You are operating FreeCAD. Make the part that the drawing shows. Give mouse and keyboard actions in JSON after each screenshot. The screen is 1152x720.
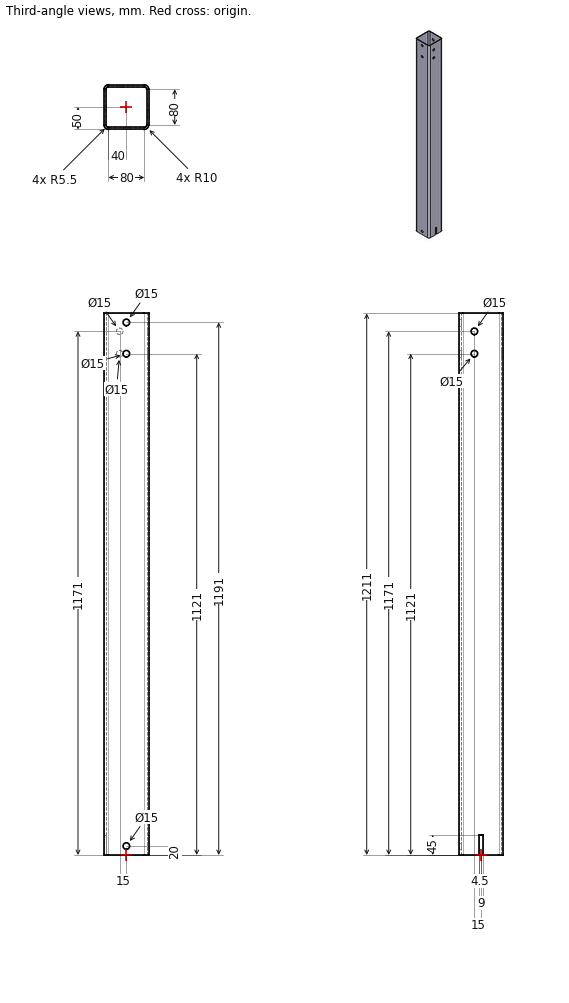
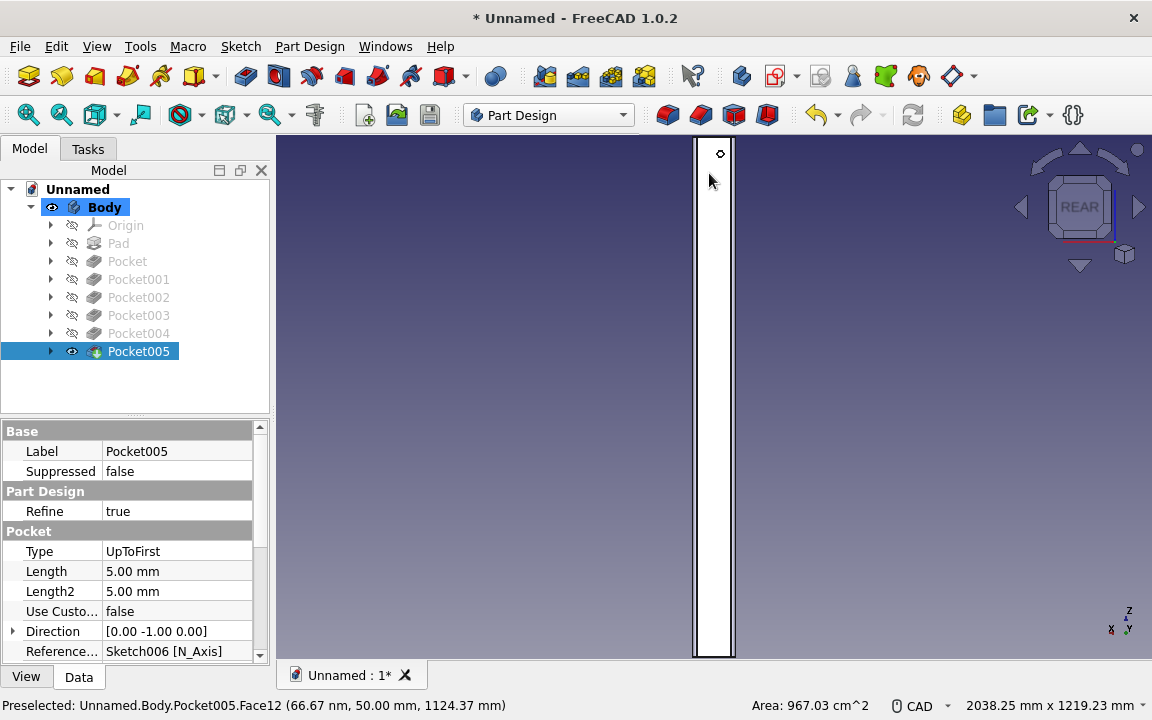
{"action": "left_click", "coordinate": [774, 76]}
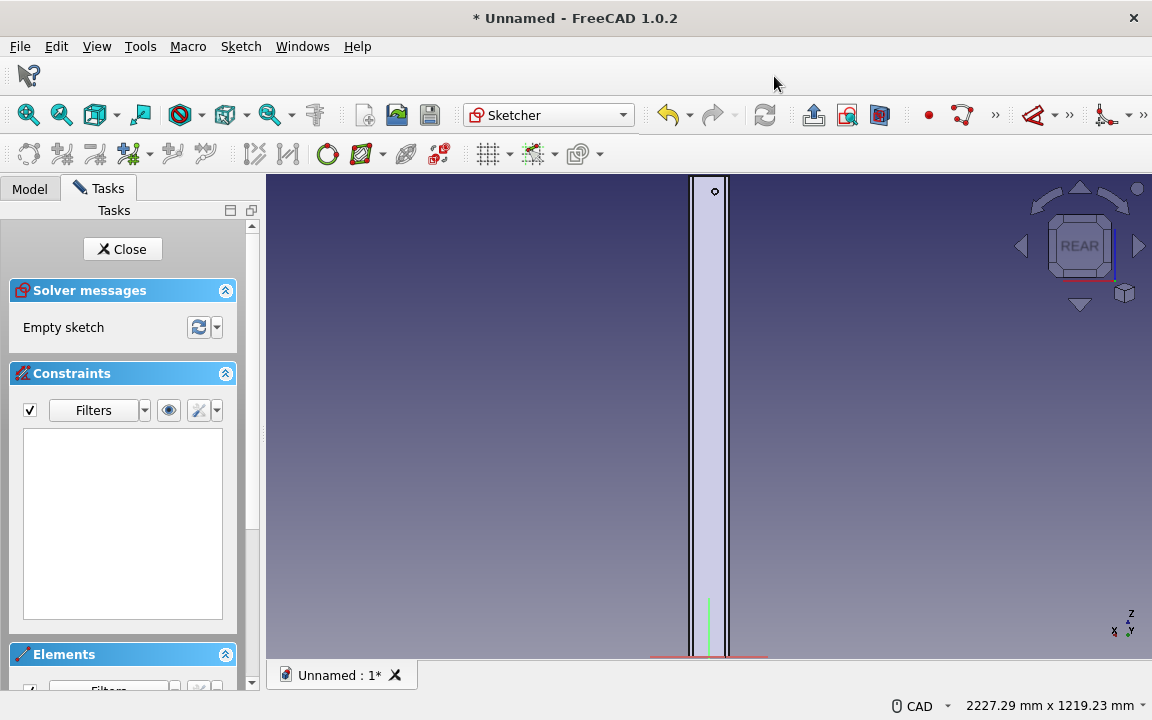
{"action": "scroll", "coordinate": [719, 202], "scroll_direction": "up", "scroll_amount": 15}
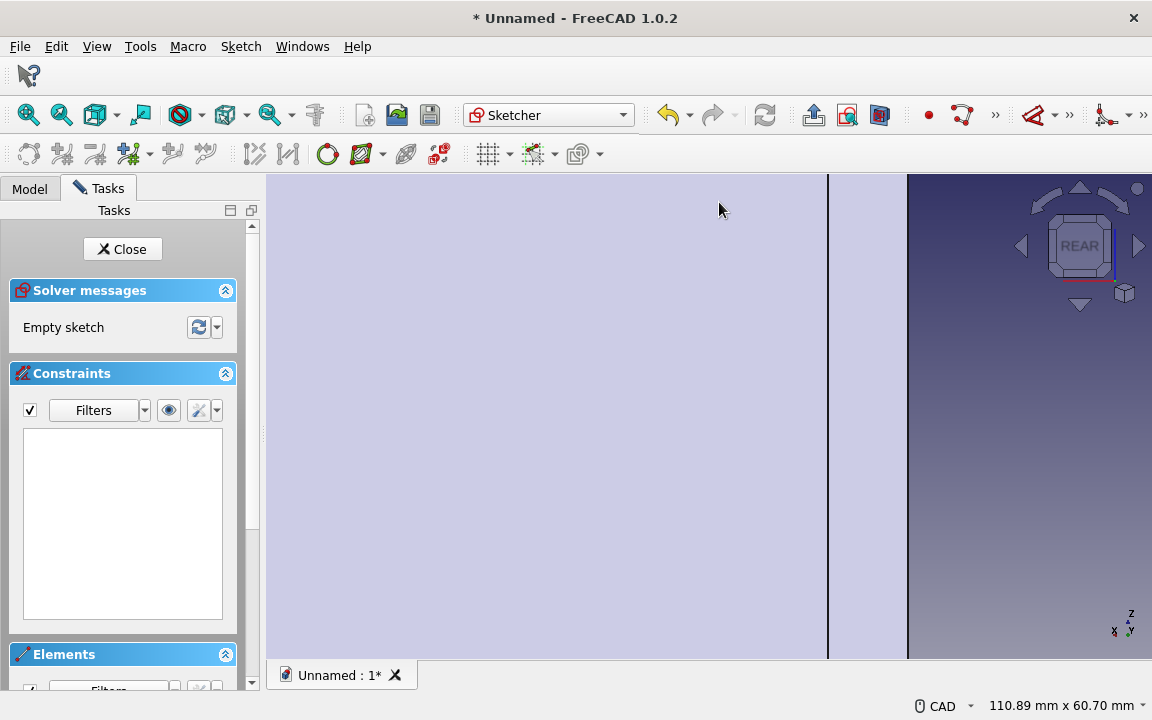
{"action": "scroll", "coordinate": [621, 375], "scroll_direction": "up", "scroll_amount": 5}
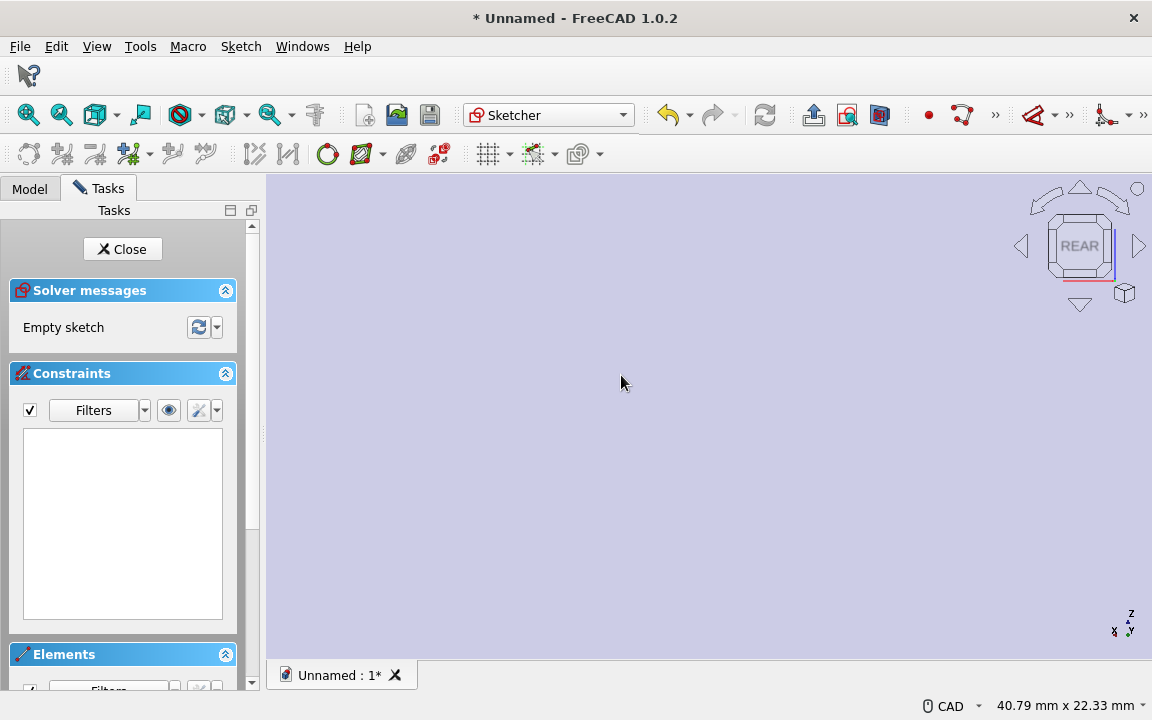
{"action": "key", "text": "g c"}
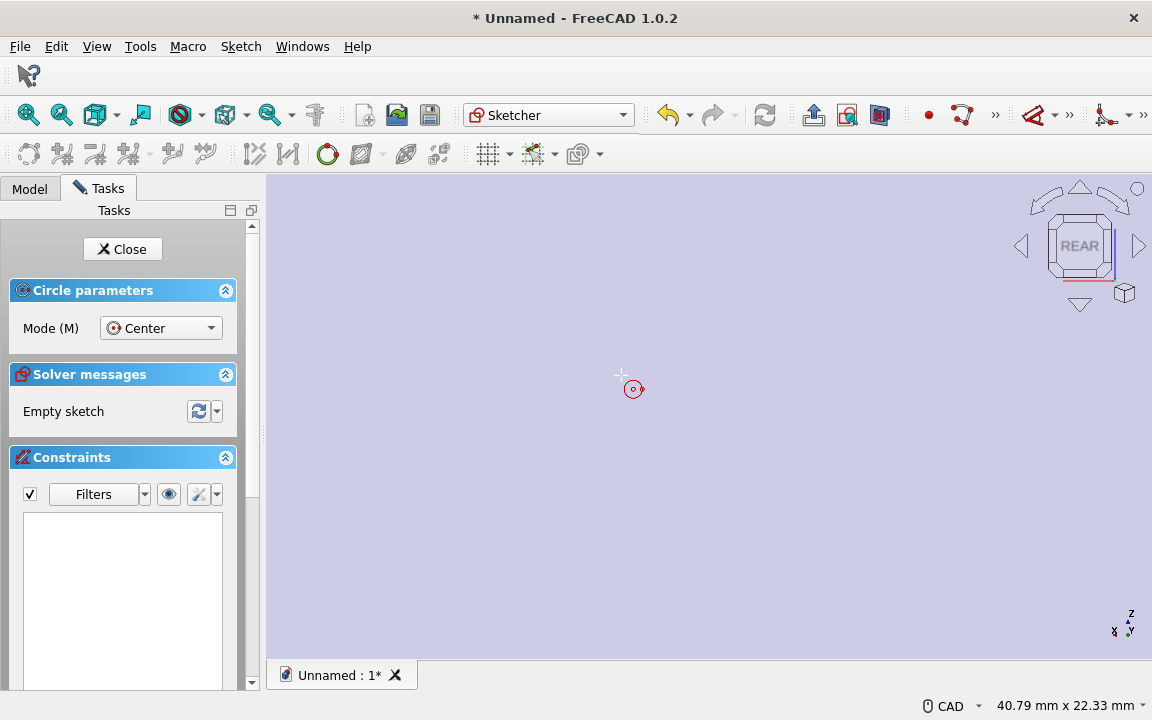
{"action": "left_click", "coordinate": [640, 416]}
{"action": "left_click", "coordinate": [755, 301]}
{"action": "key", "text": "Escape"}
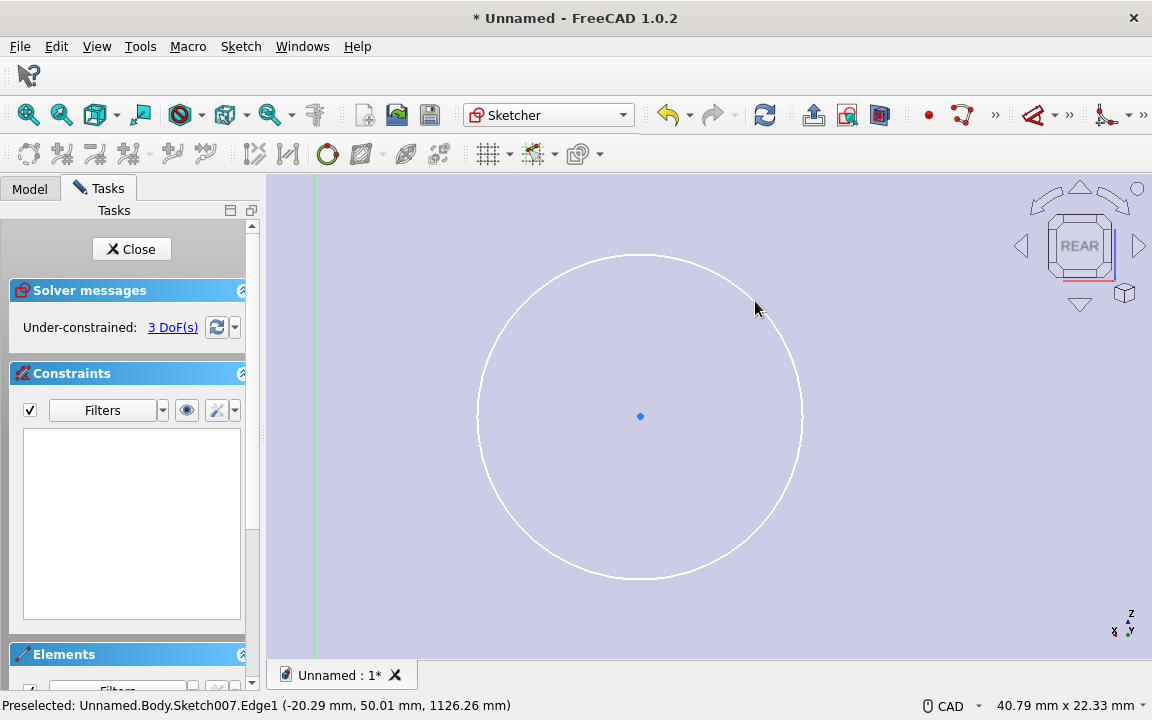
{"action": "key", "text": "d"}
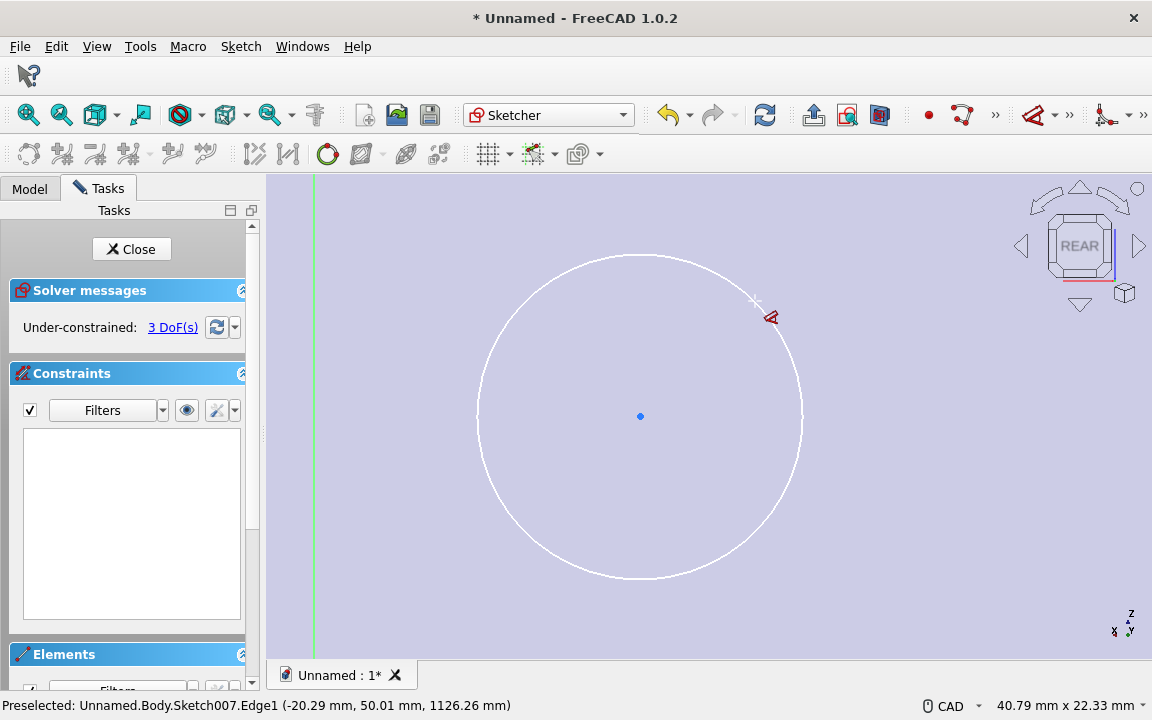
{"action": "left_click", "coordinate": [755, 302]}
{"action": "left_click", "coordinate": [778, 279]}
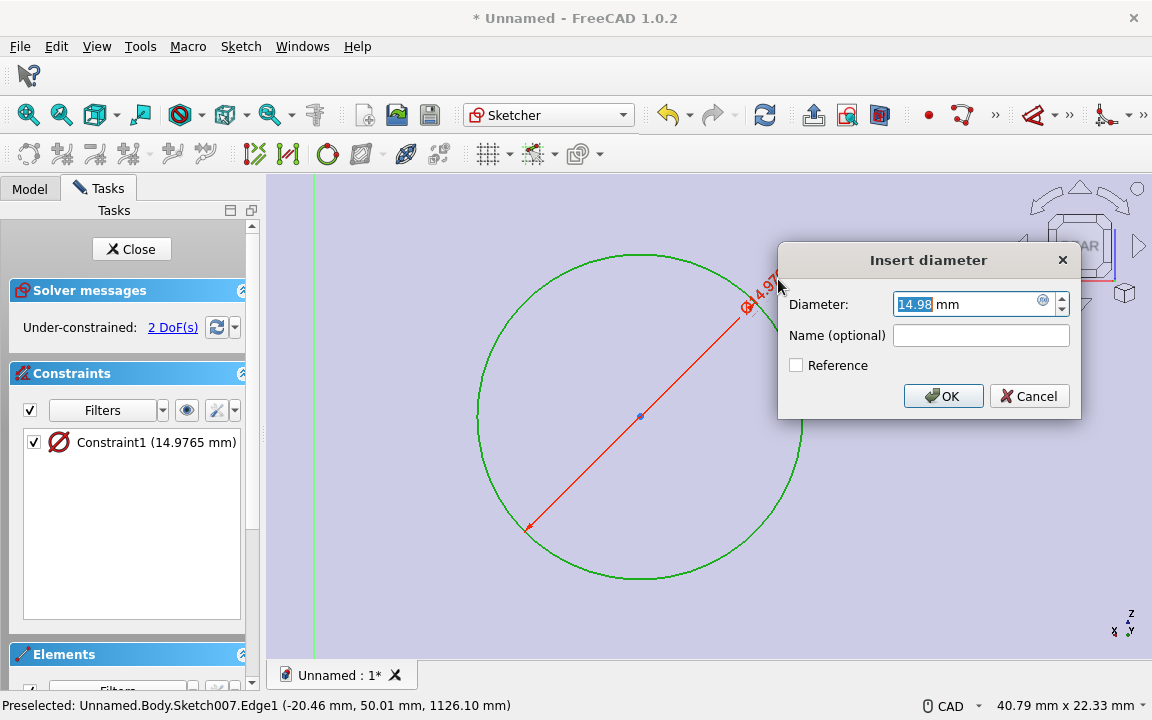
{"action": "type", "text": "15"}
{"action": "key", "text": "Return"}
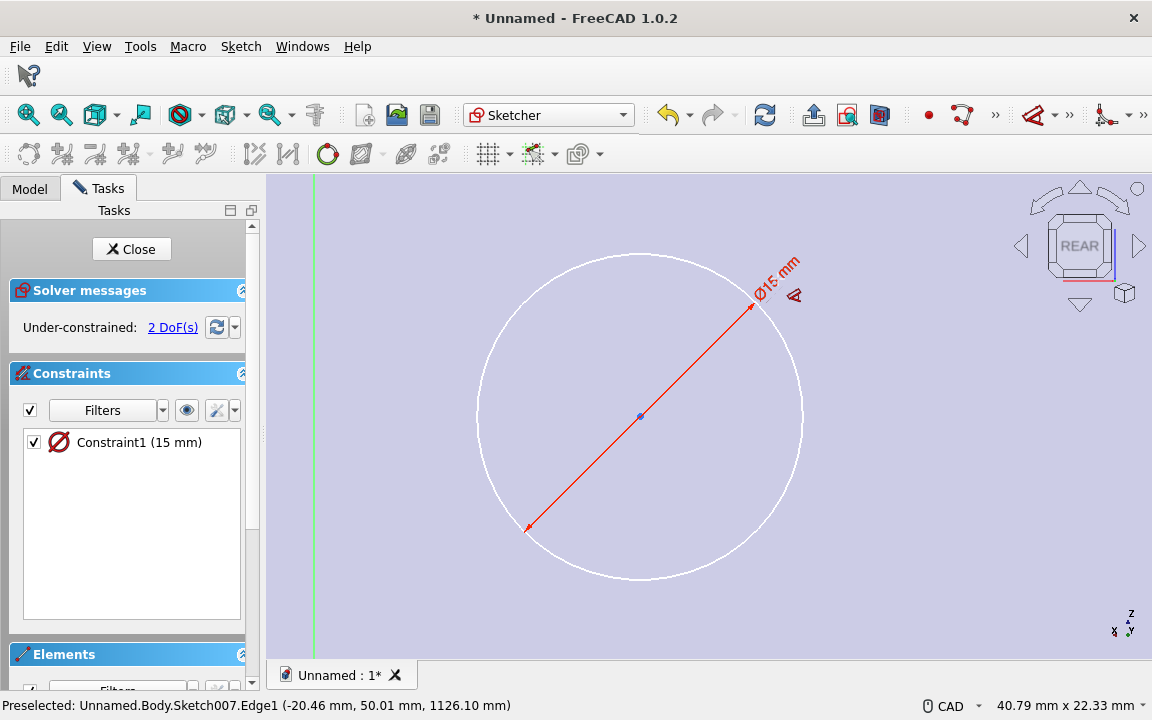
{"action": "left_click", "coordinate": [640, 417]}
{"action": "left_click", "coordinate": [402, 383]}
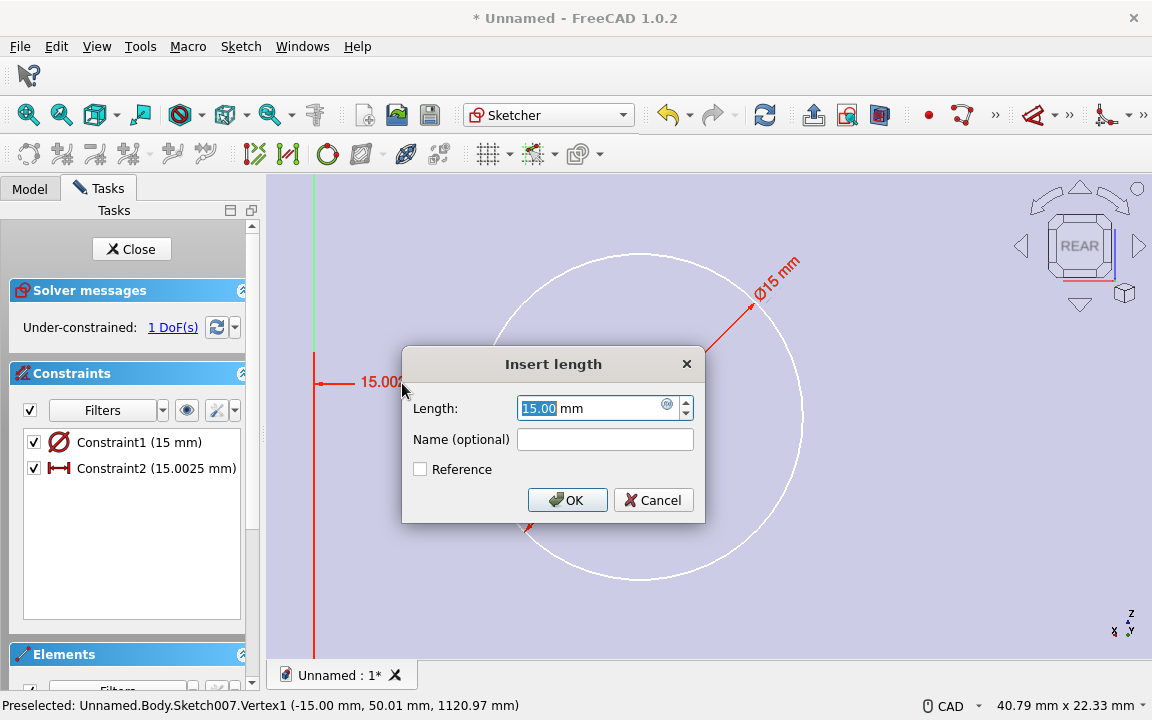
{"action": "type", "text": "15"}
{"action": "key", "text": "Return"}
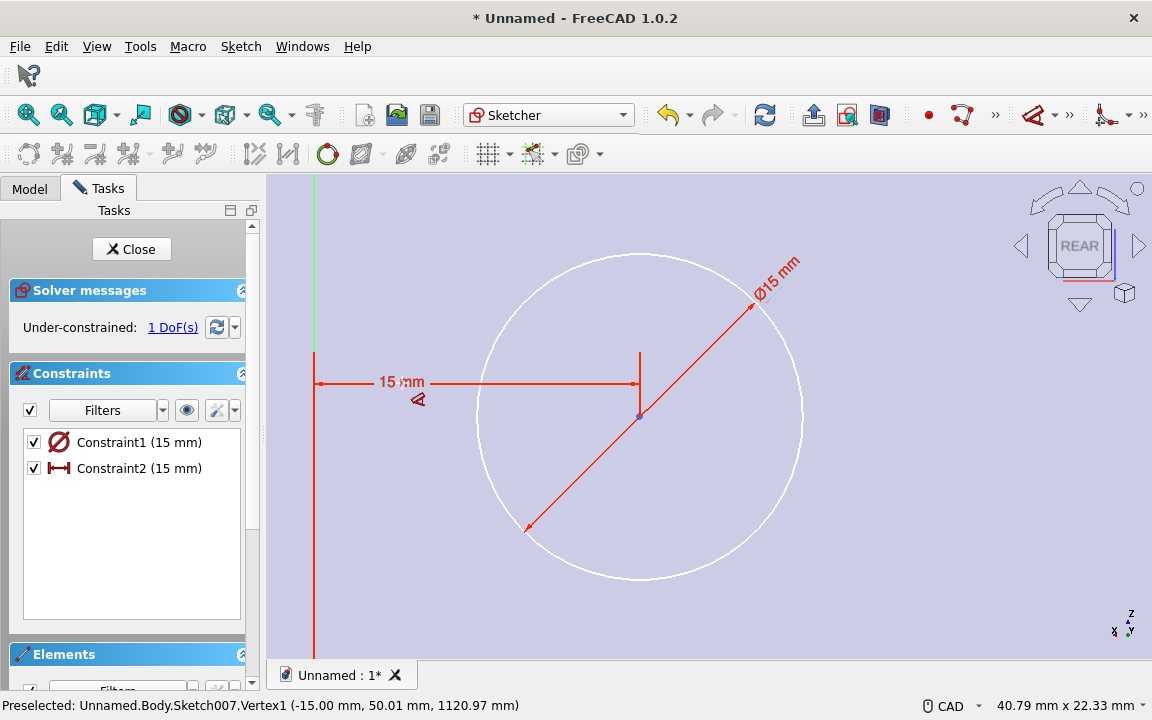
{"action": "left_click", "coordinate": [640, 417]}
{"action": "left_click", "coordinate": [674, 524]}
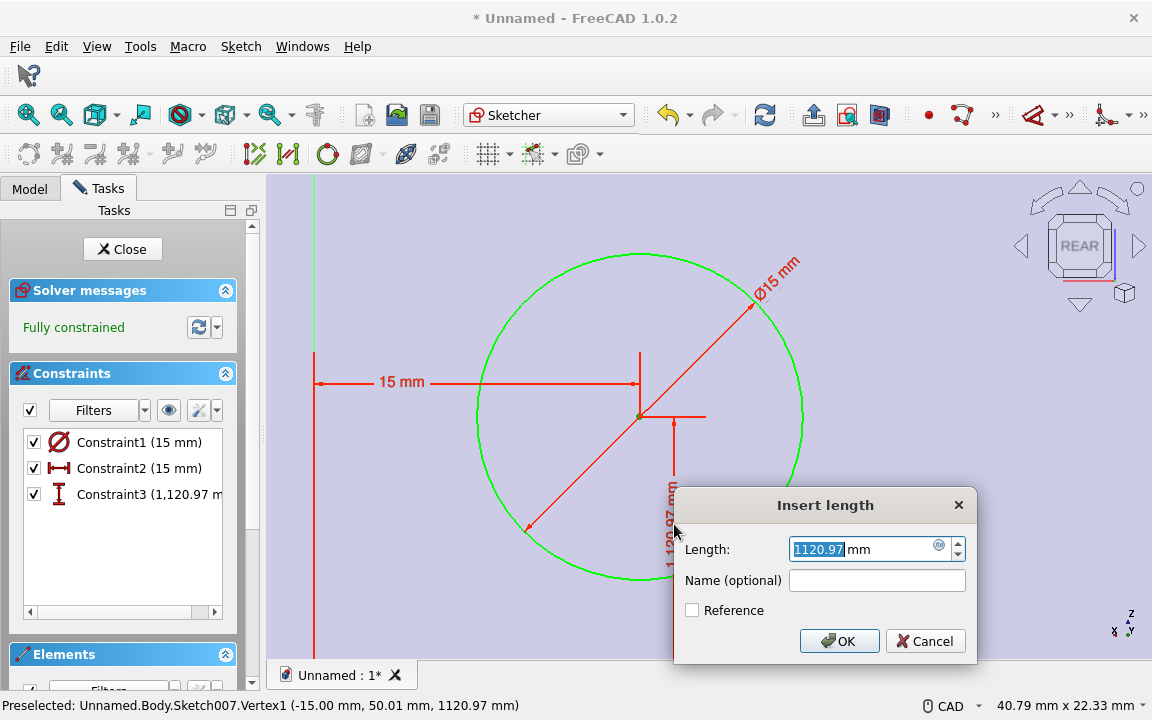
{"action": "type", "text": "1121"}
{"action": "key", "text": "Return"}
{"action": "key", "text": "Escape"}